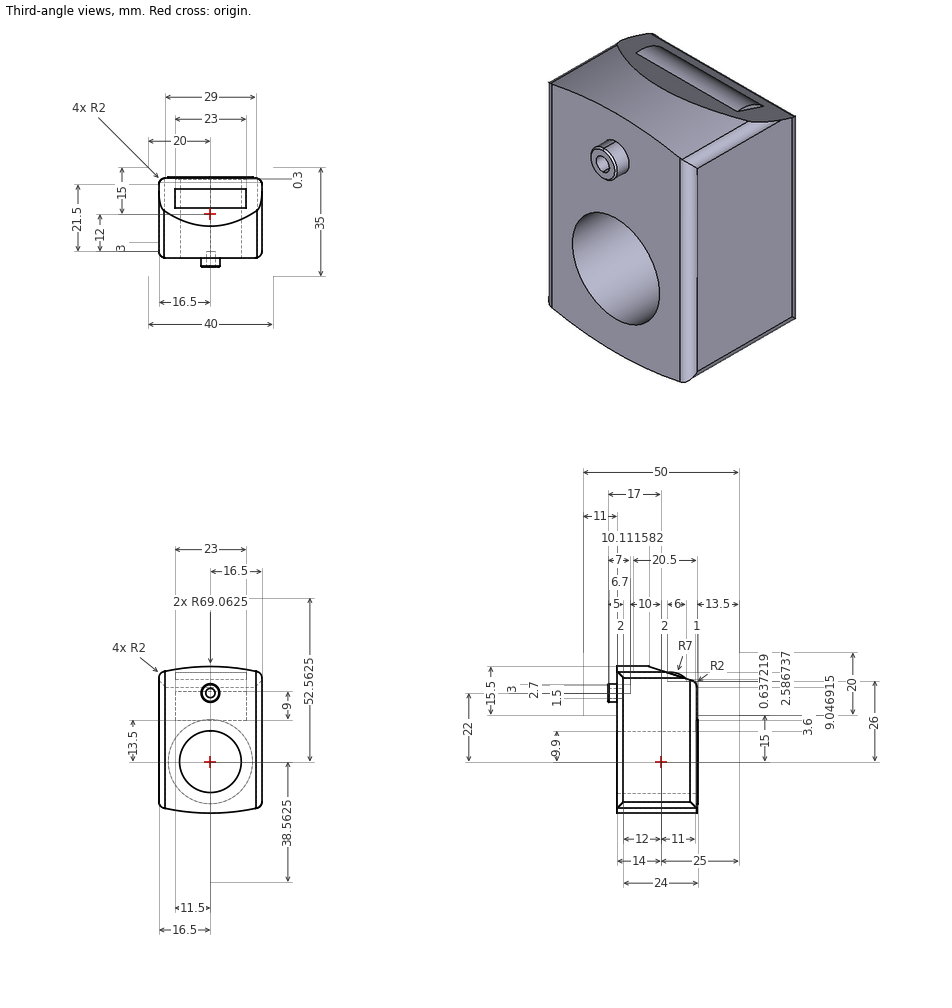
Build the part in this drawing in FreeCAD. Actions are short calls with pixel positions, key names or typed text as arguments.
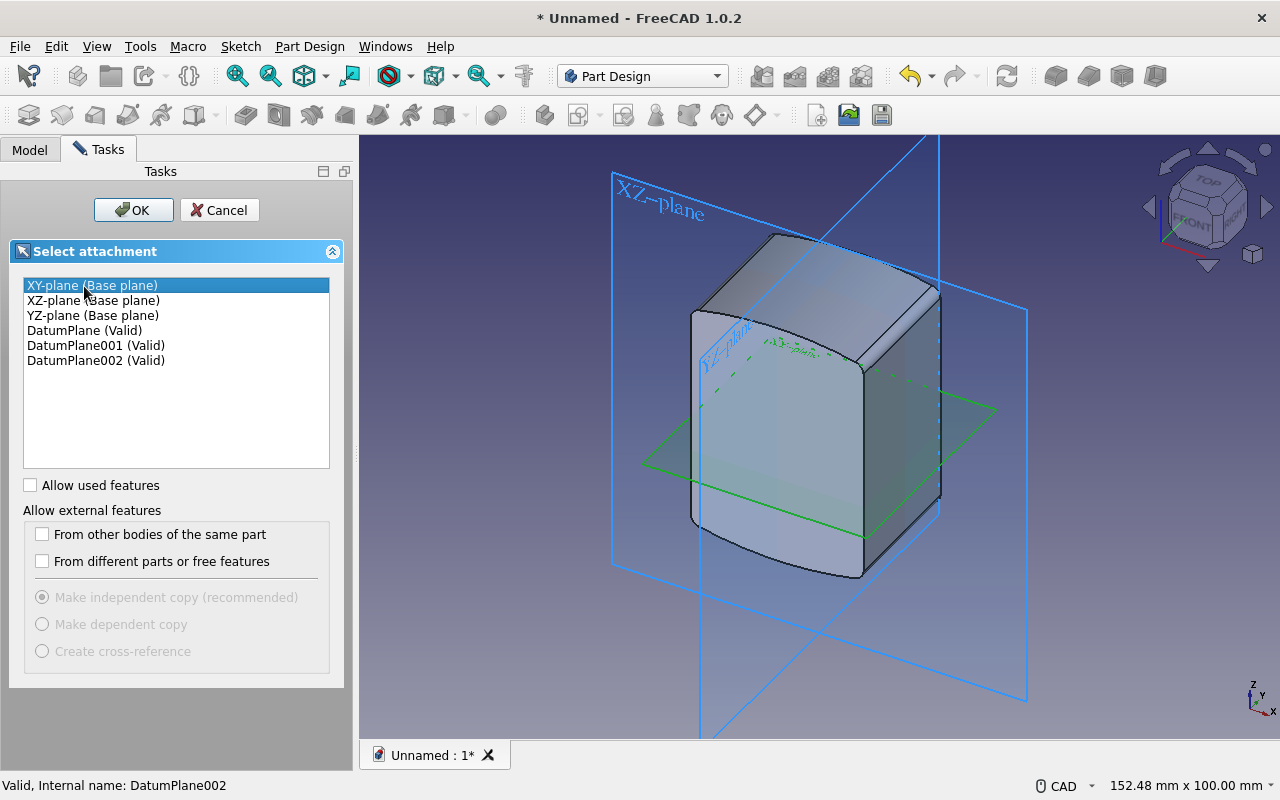
click(134, 210)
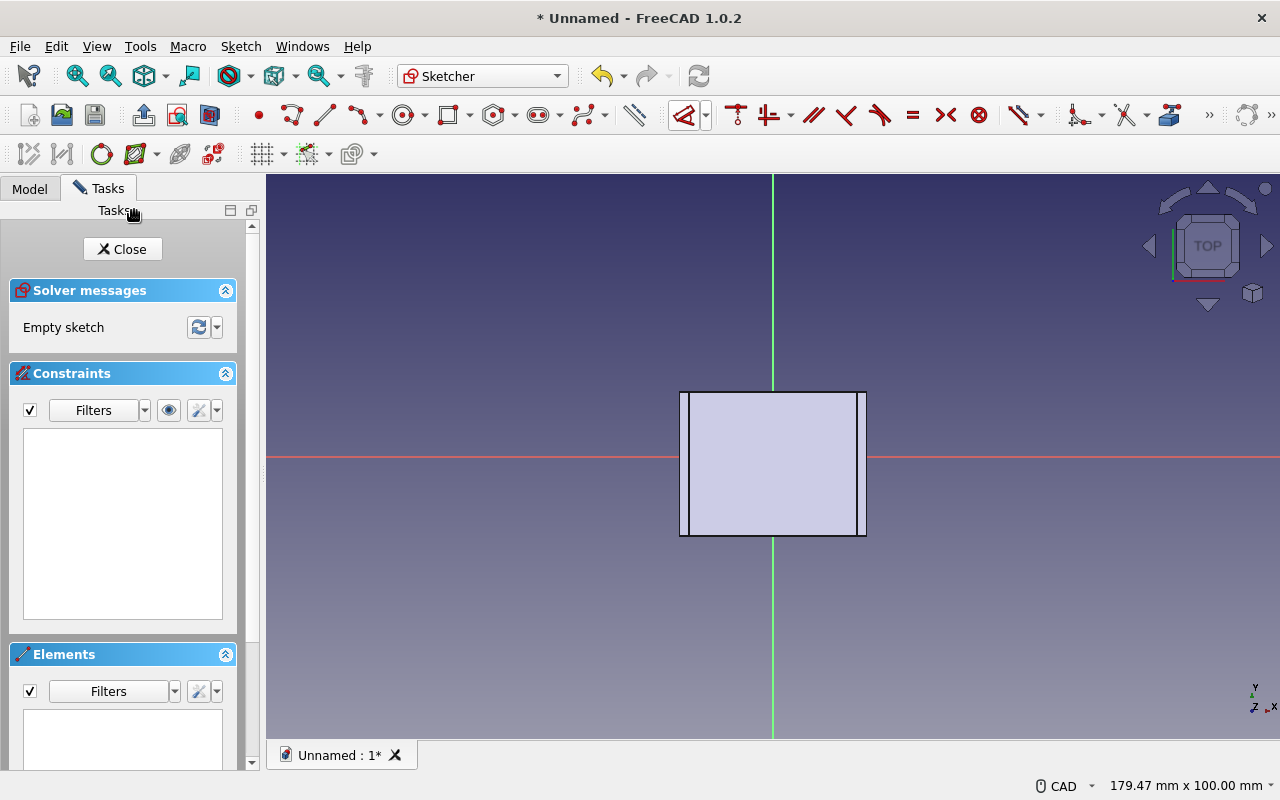
click(210, 116)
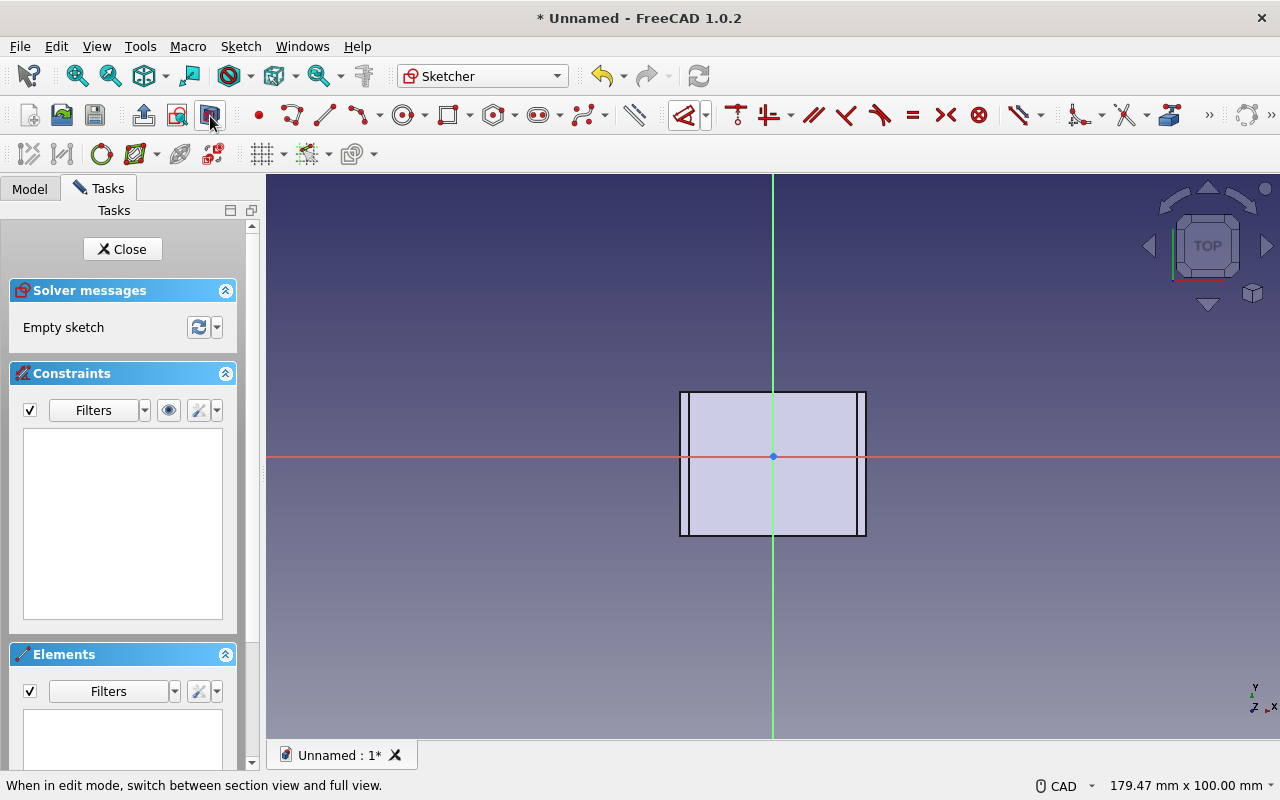
scroll(856, 488, up, 3)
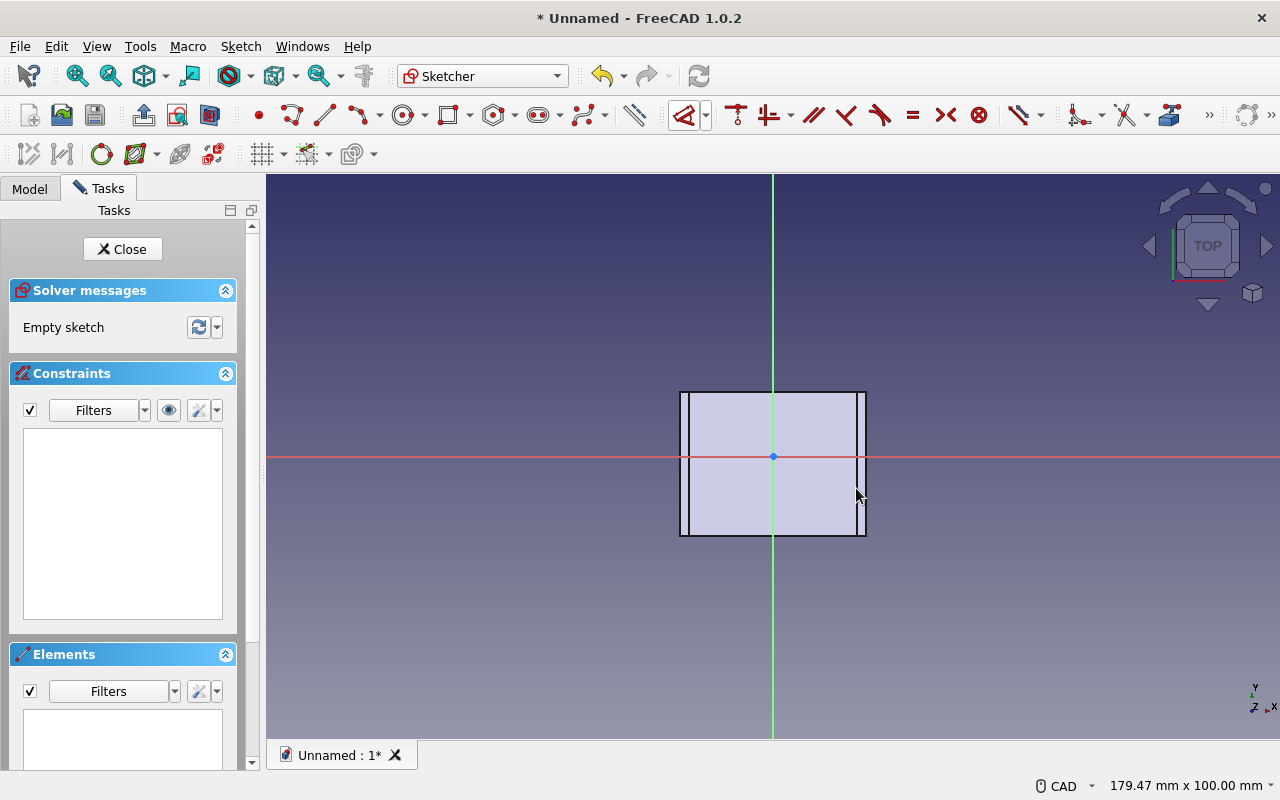
click(448, 116)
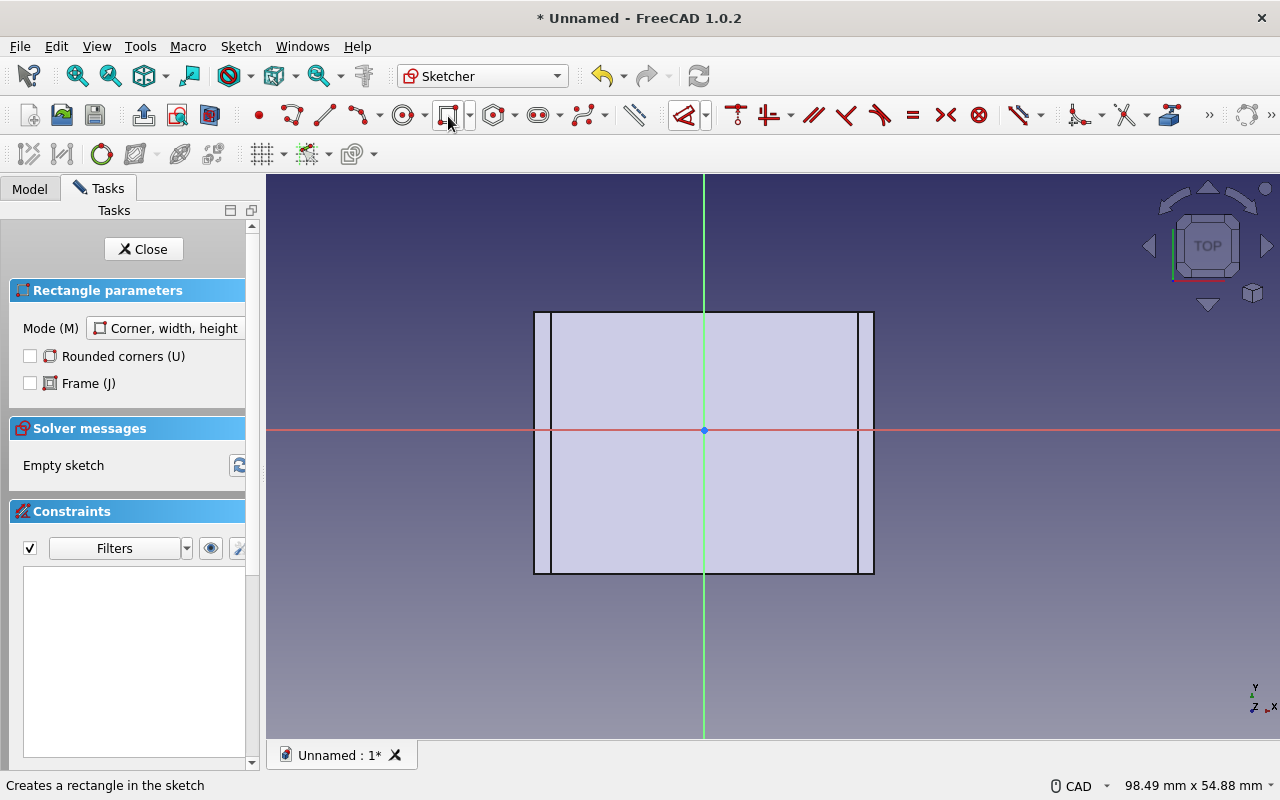
click(498, 276)
move(910, 636)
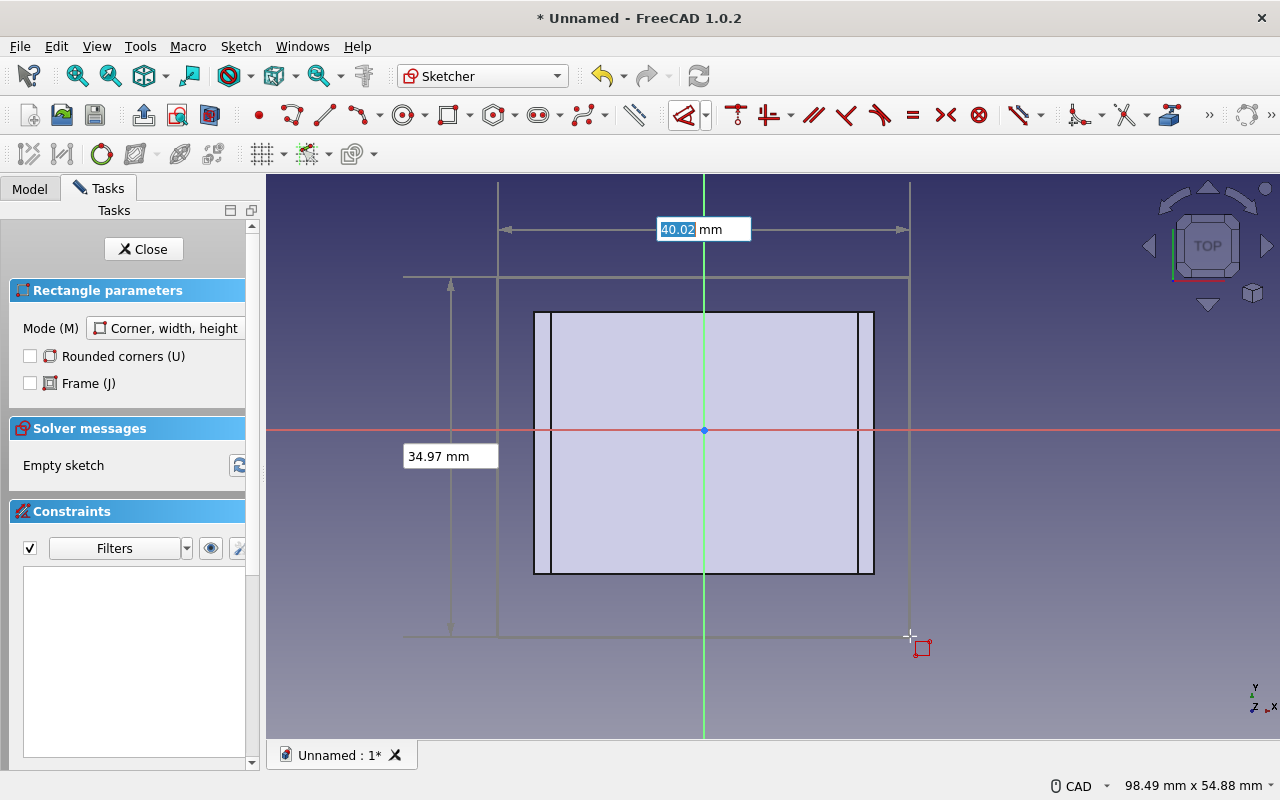
text(40)
key(Tab)
text(35)
key(Return)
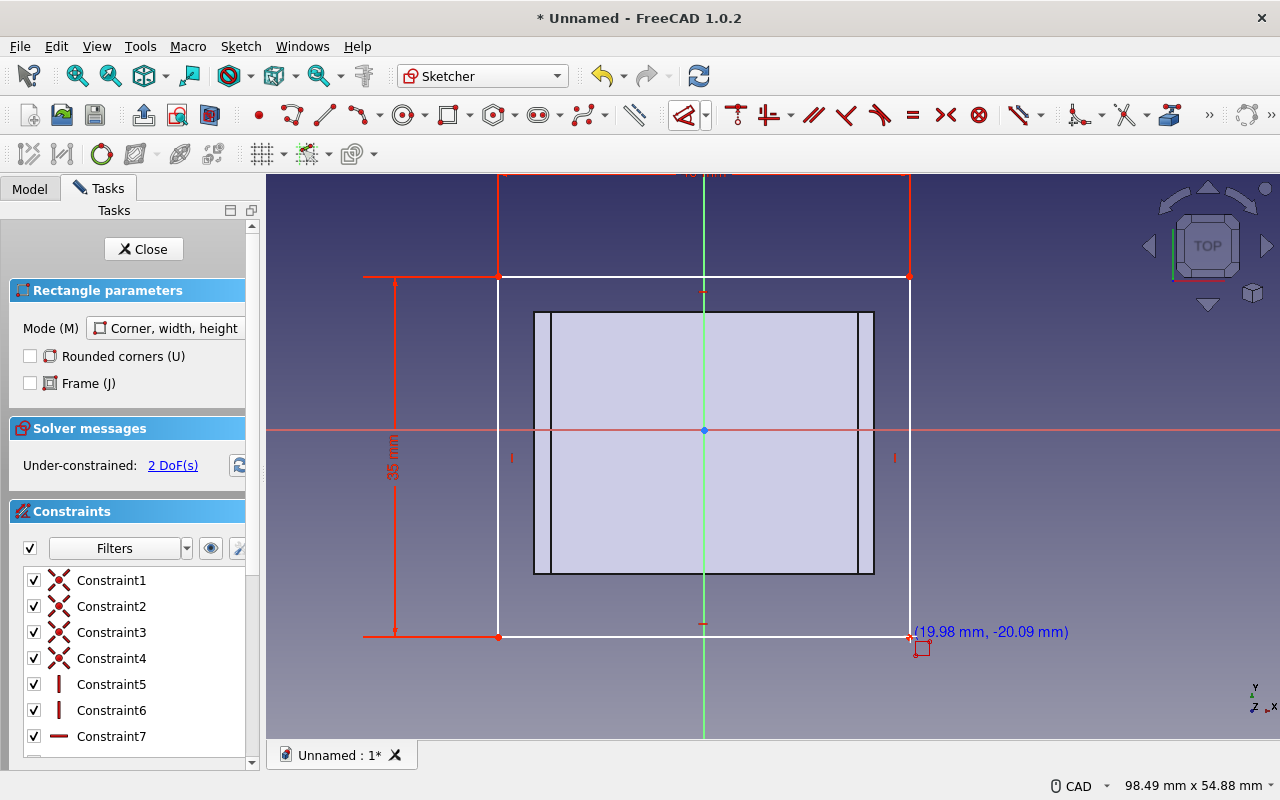
click(325, 116)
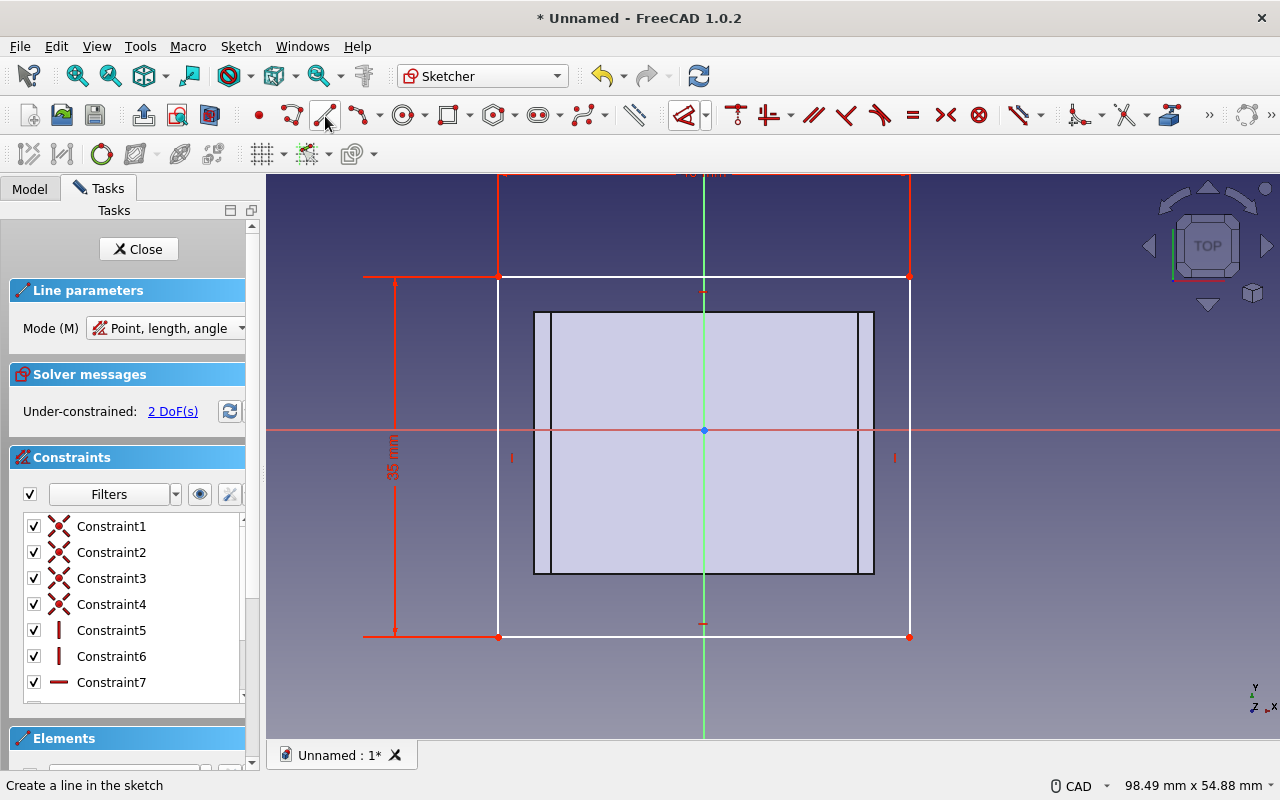
click(534, 554)
click(534, 332)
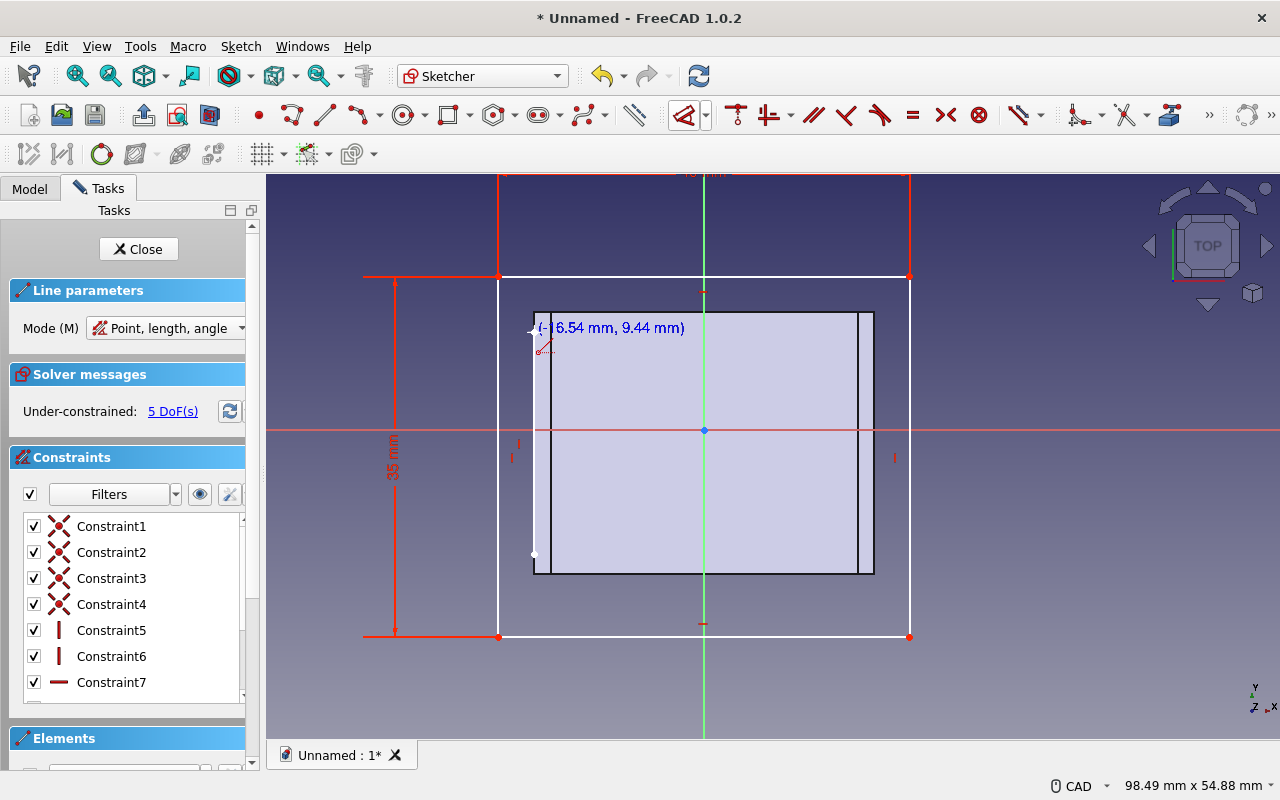
click(555, 312)
click(854, 312)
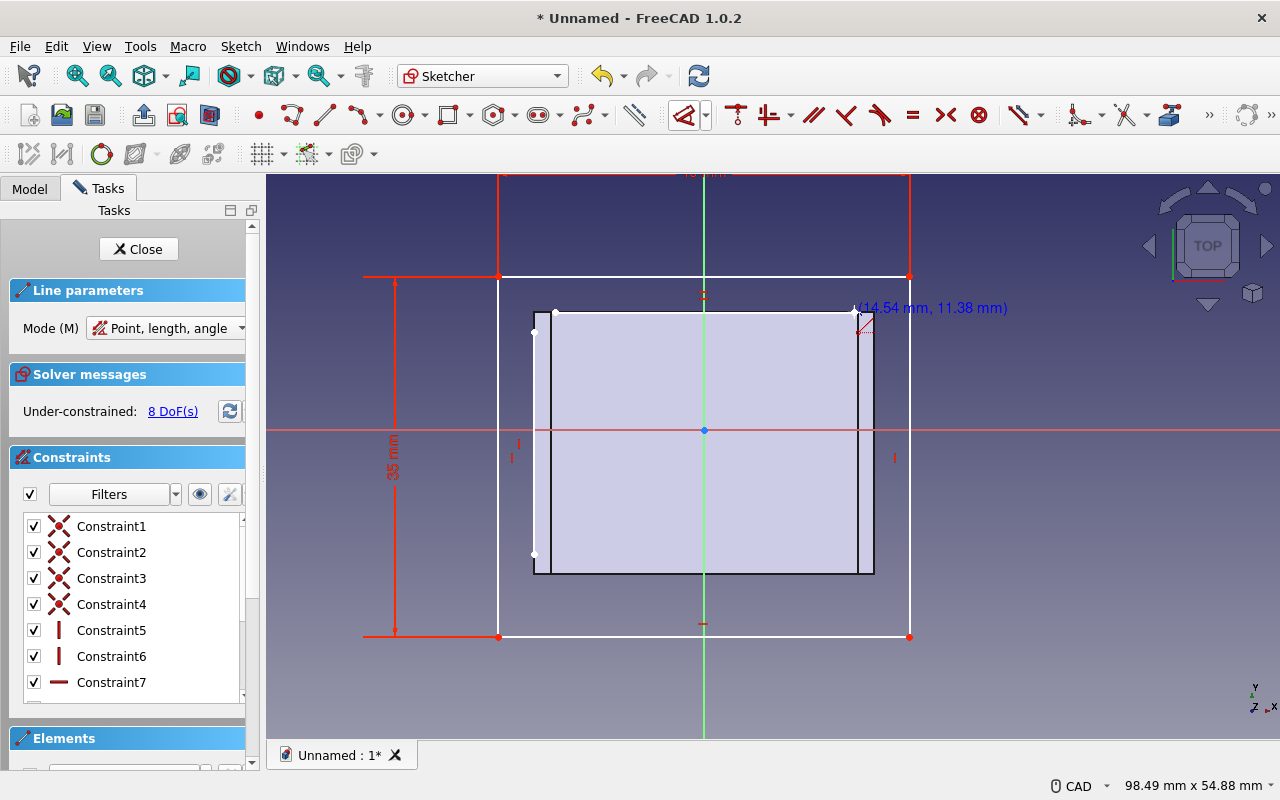
click(874, 332)
click(874, 554)